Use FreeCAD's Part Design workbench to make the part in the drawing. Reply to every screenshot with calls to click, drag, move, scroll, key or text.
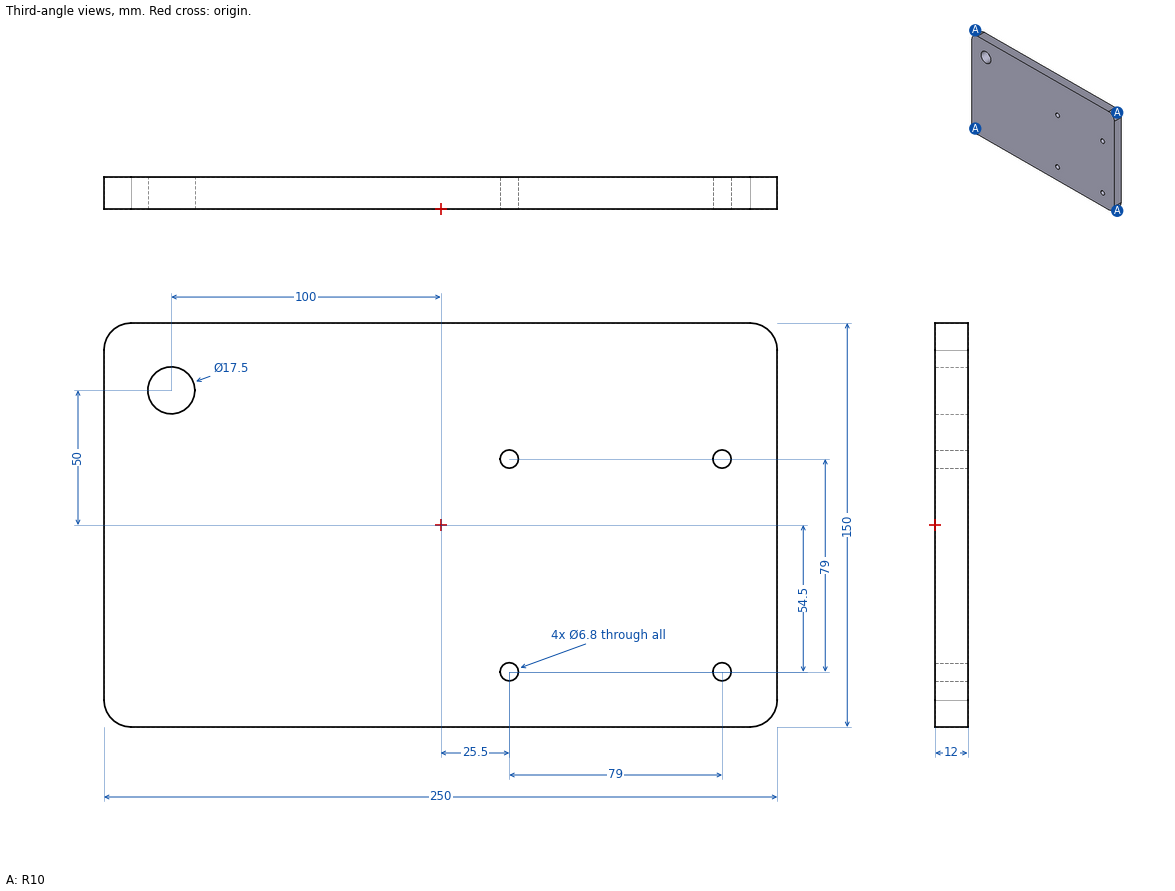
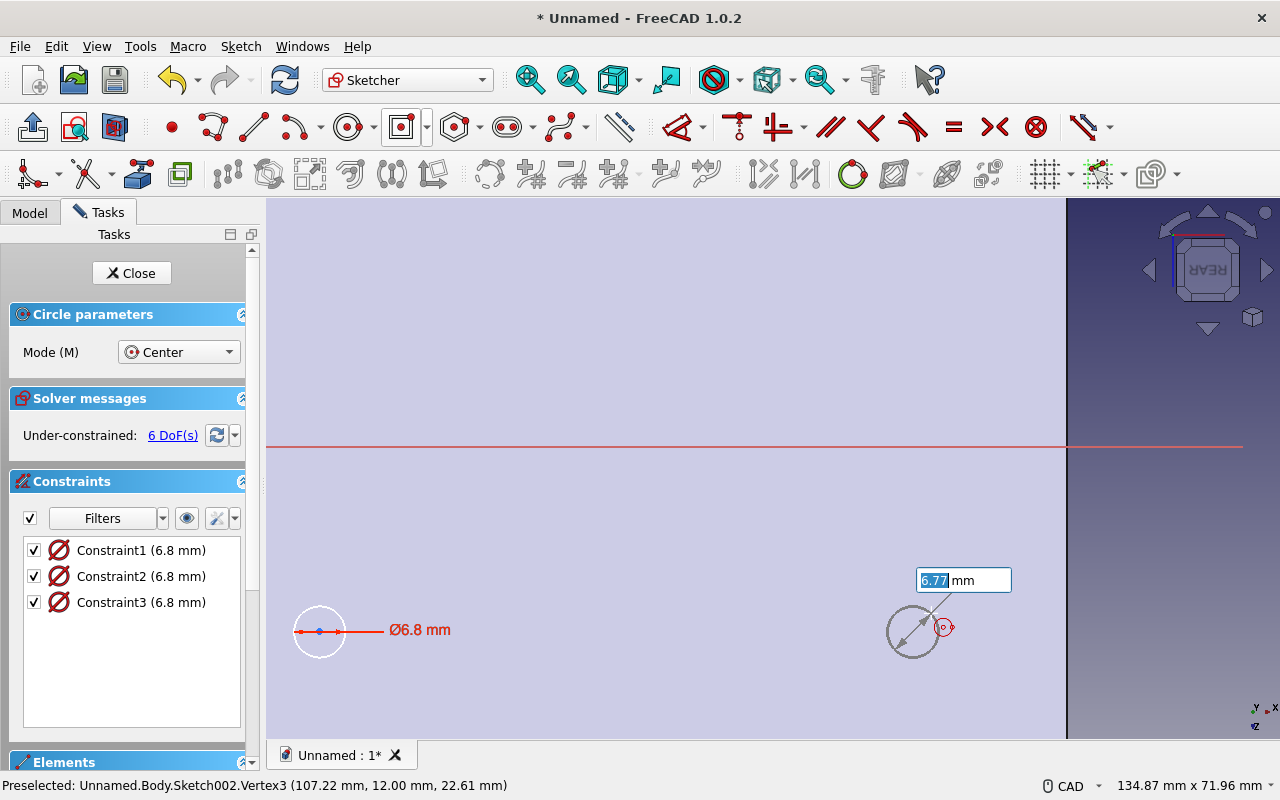
text(6.8)
key(Return)
key(Escape)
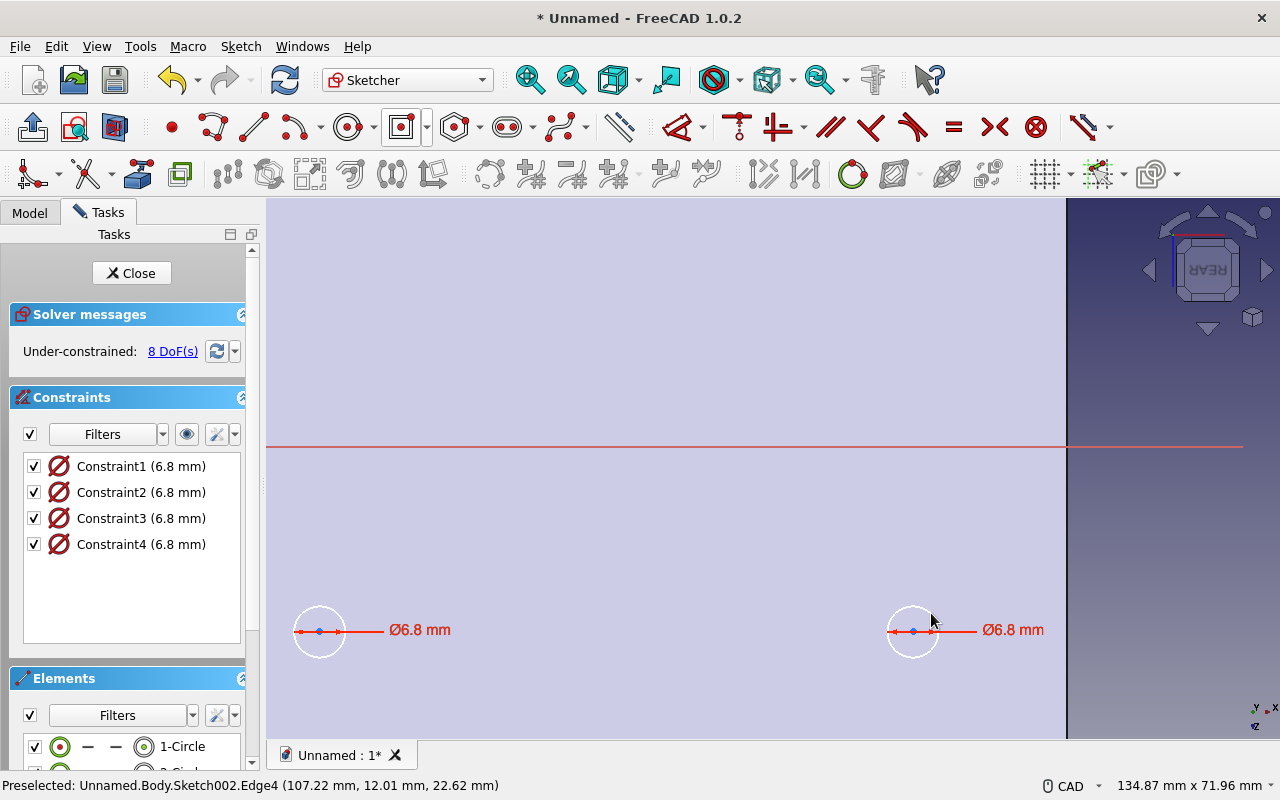
scroll(913, 632, down, 3)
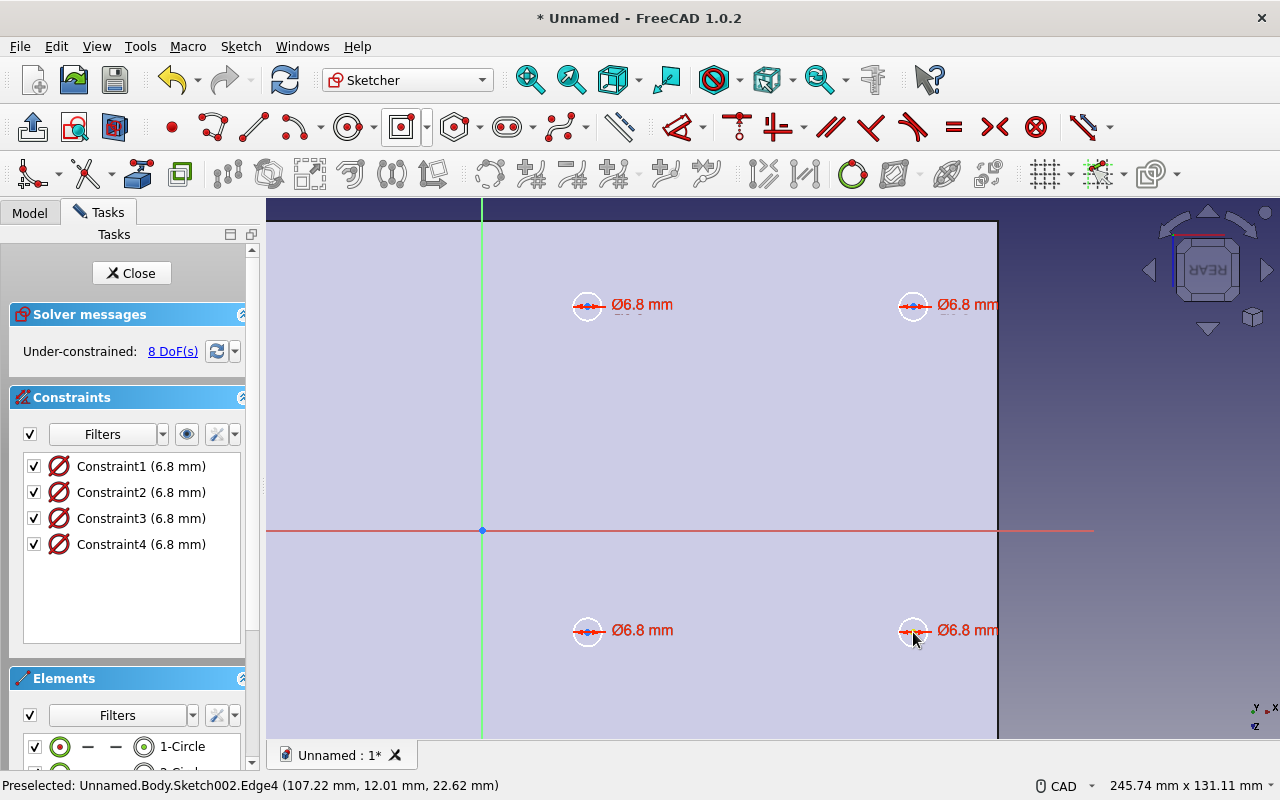
click(587, 307)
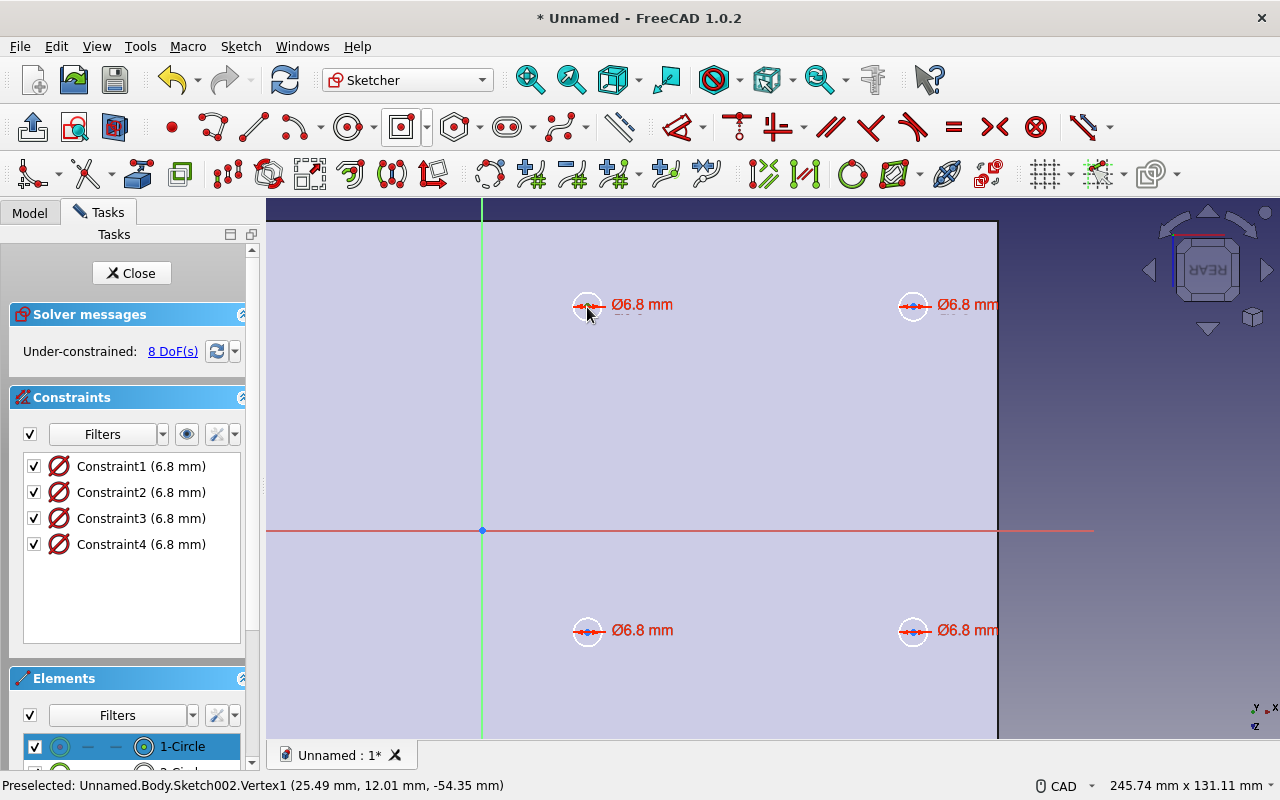
click(913, 307)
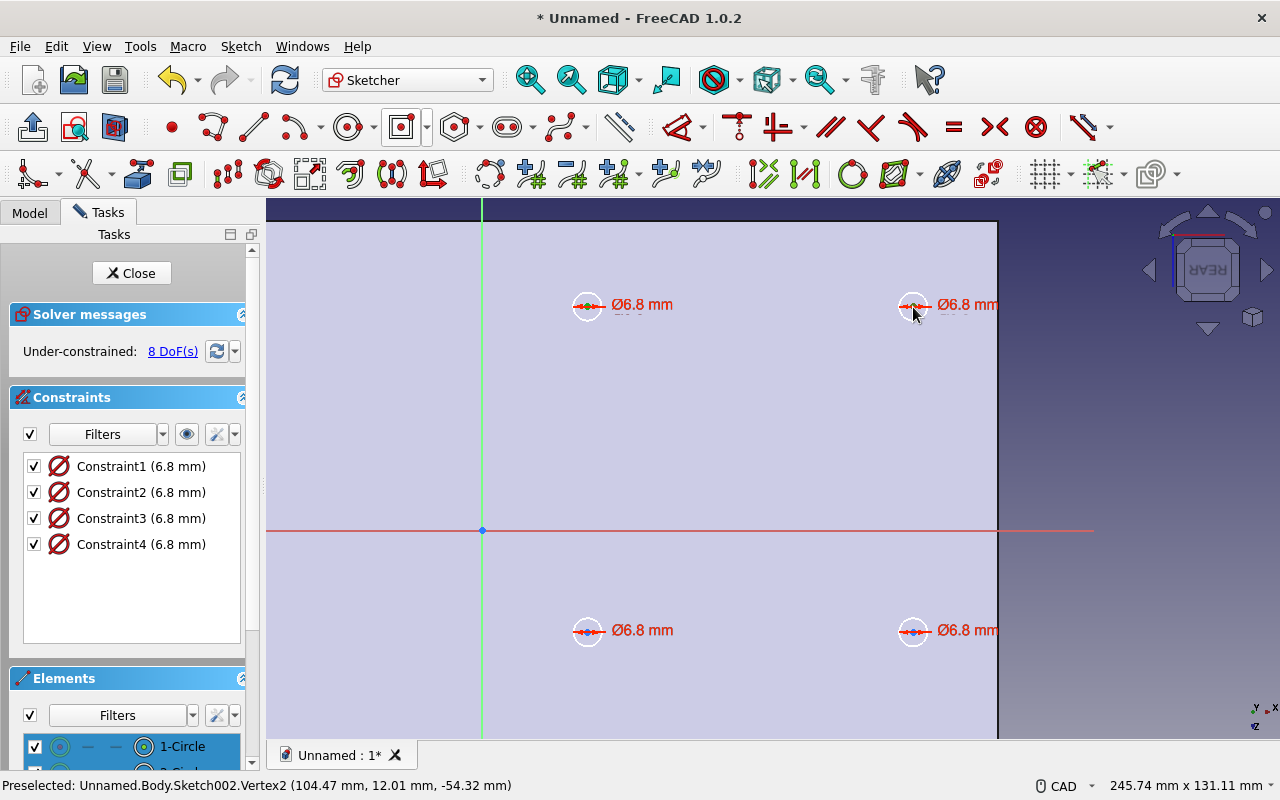
click(804, 128)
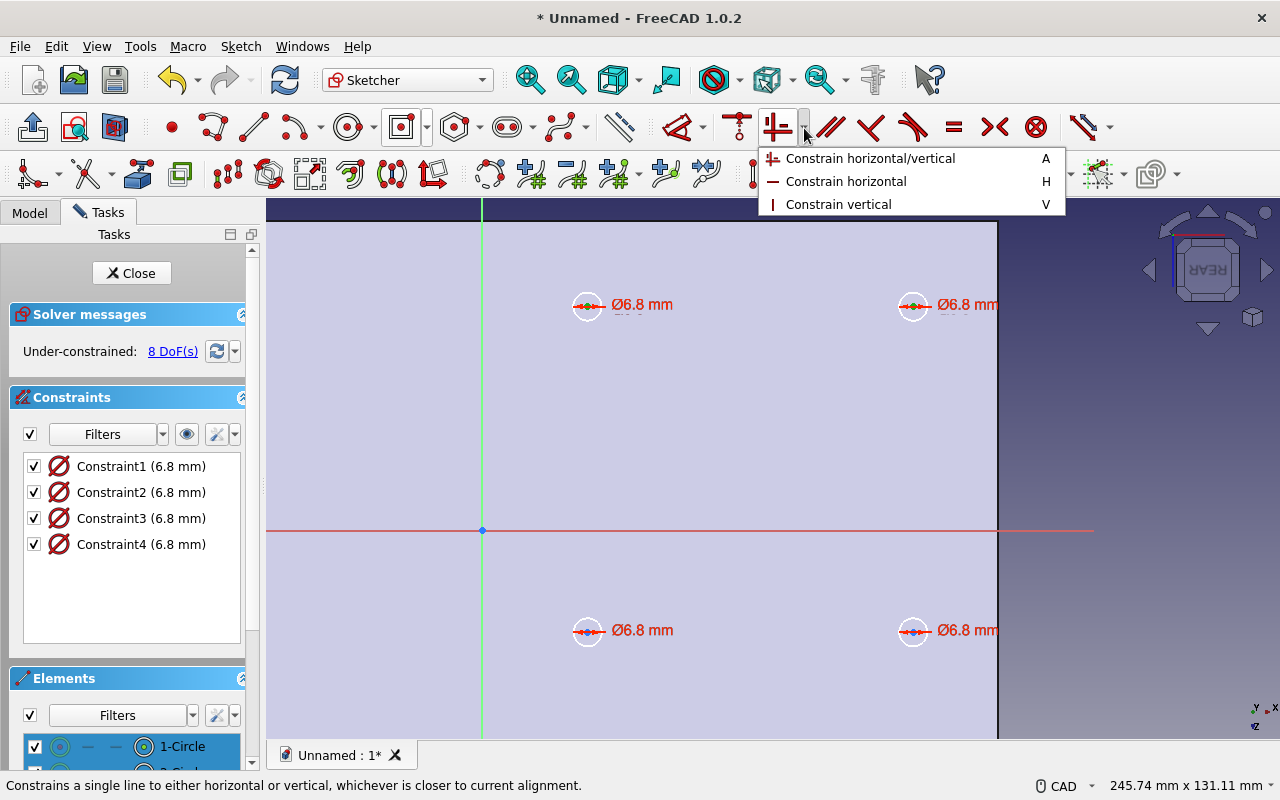
click(912, 182)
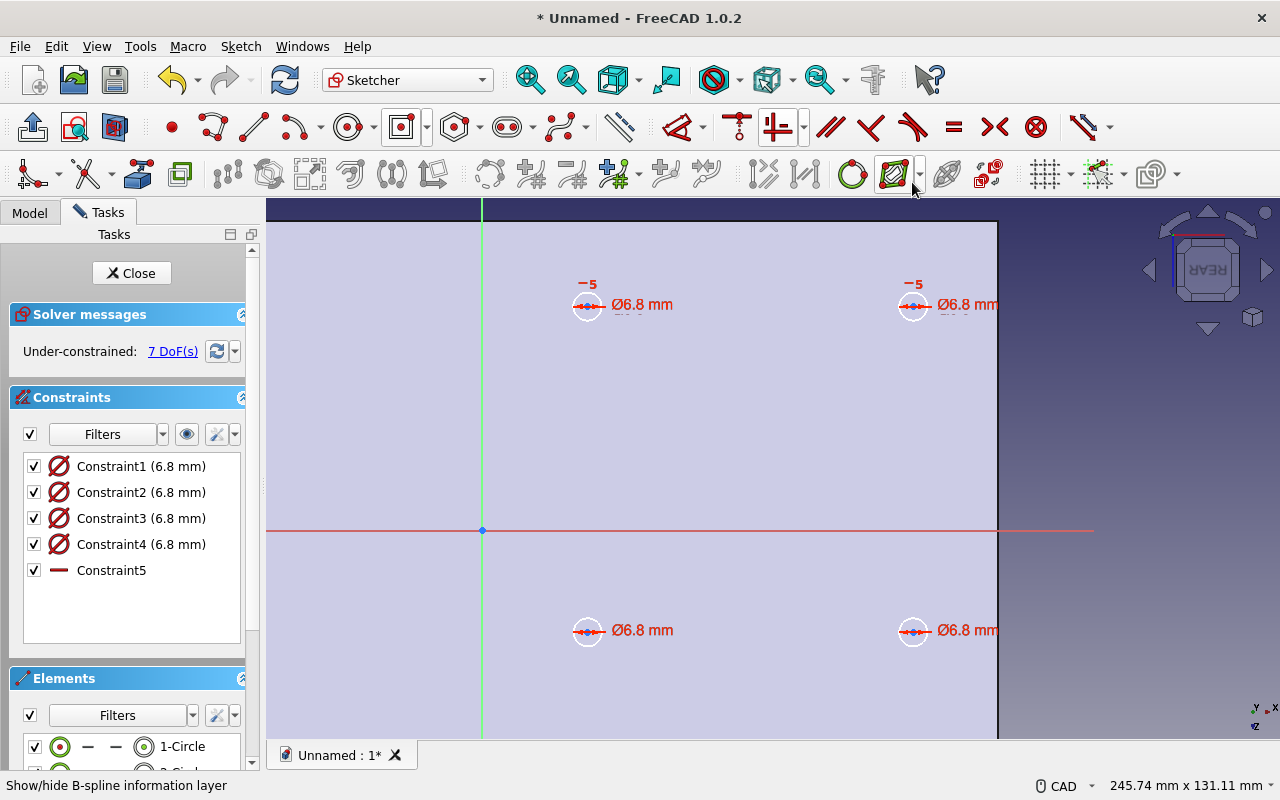
click(587, 307)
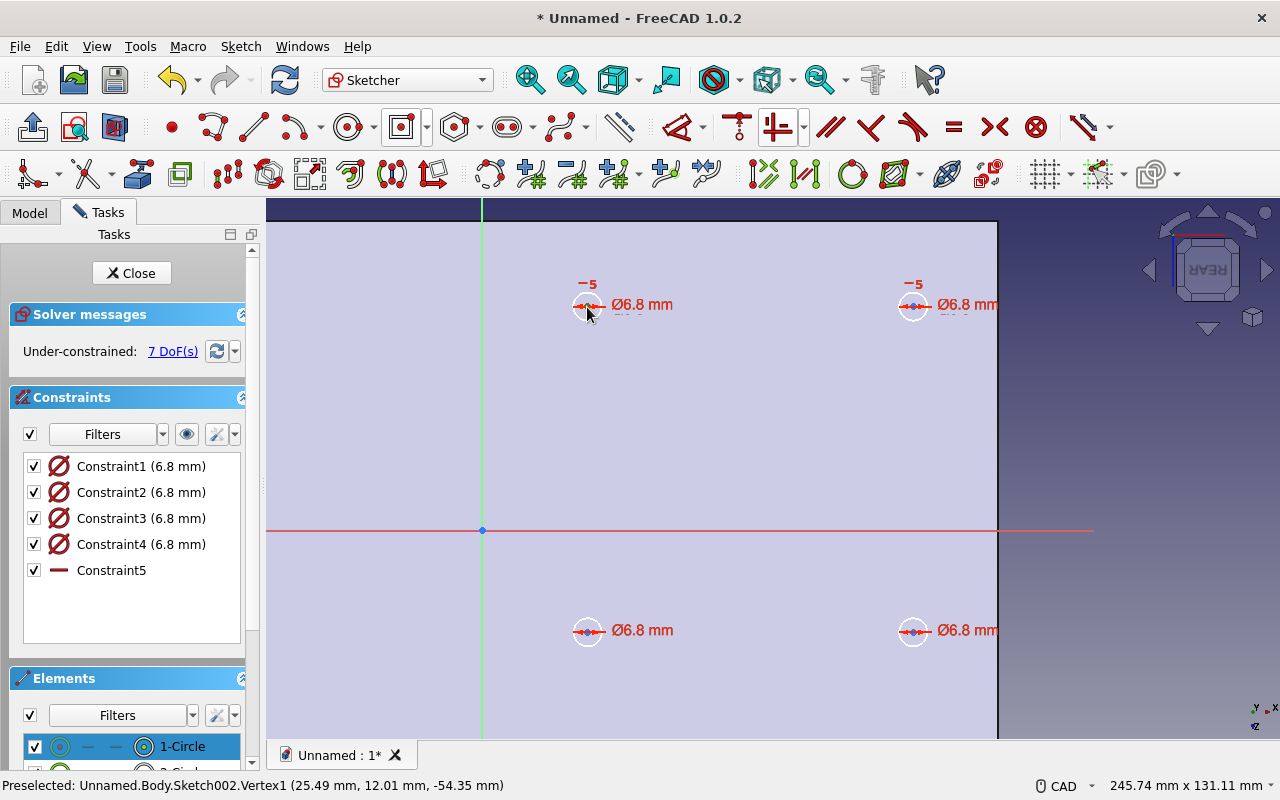
click(588, 632)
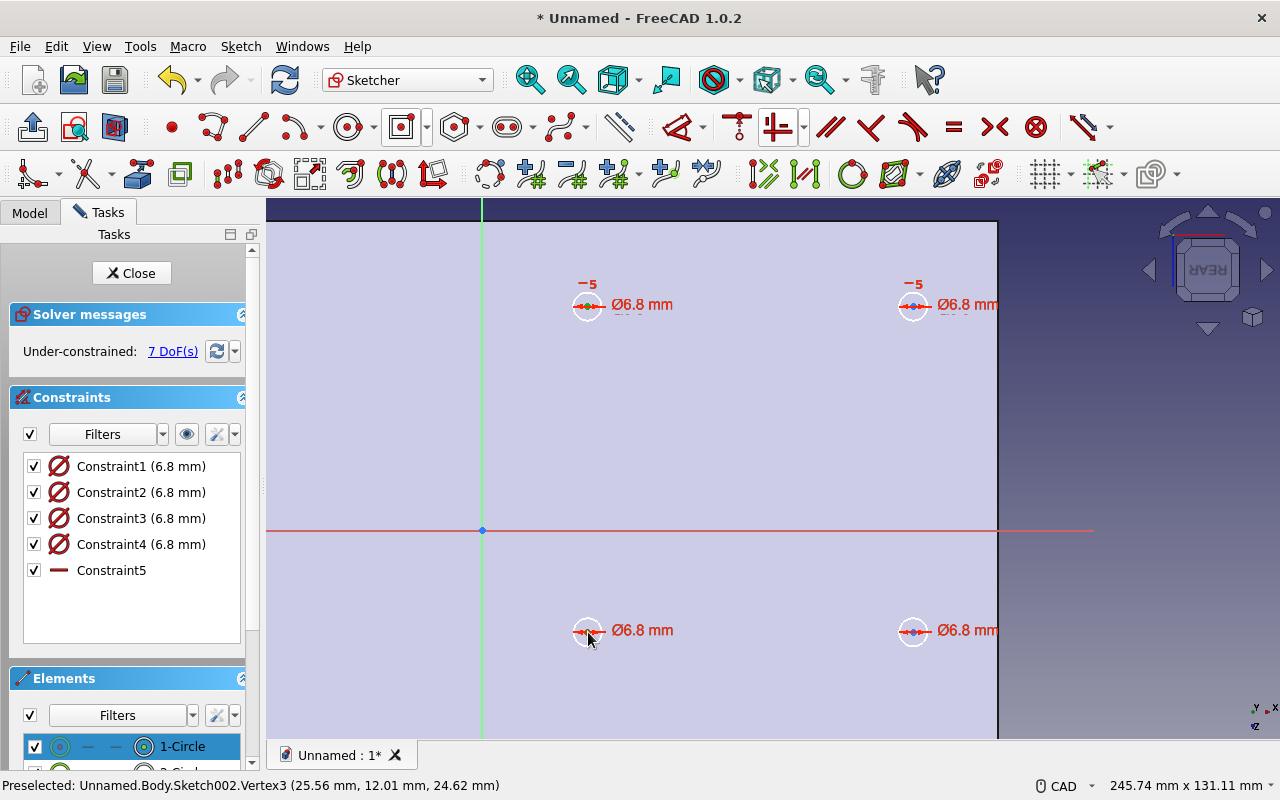
click(804, 128)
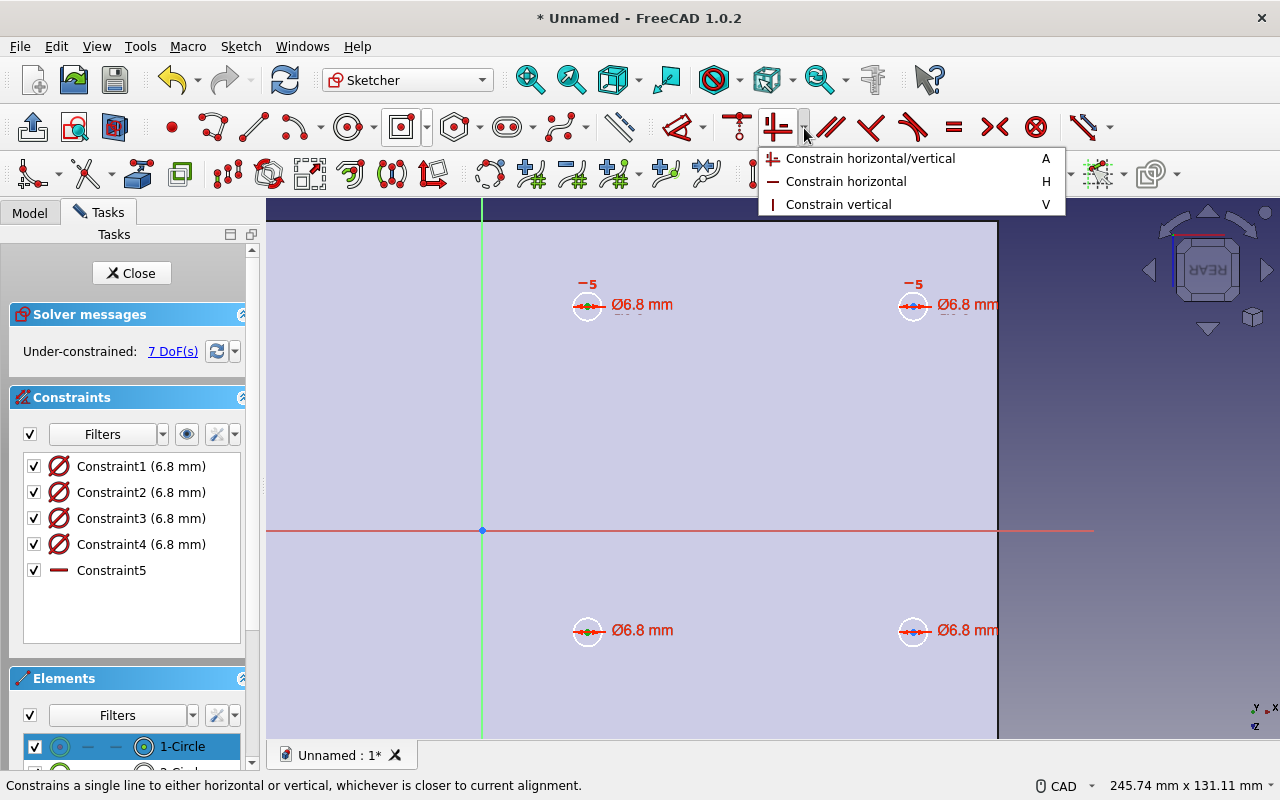
click(912, 204)